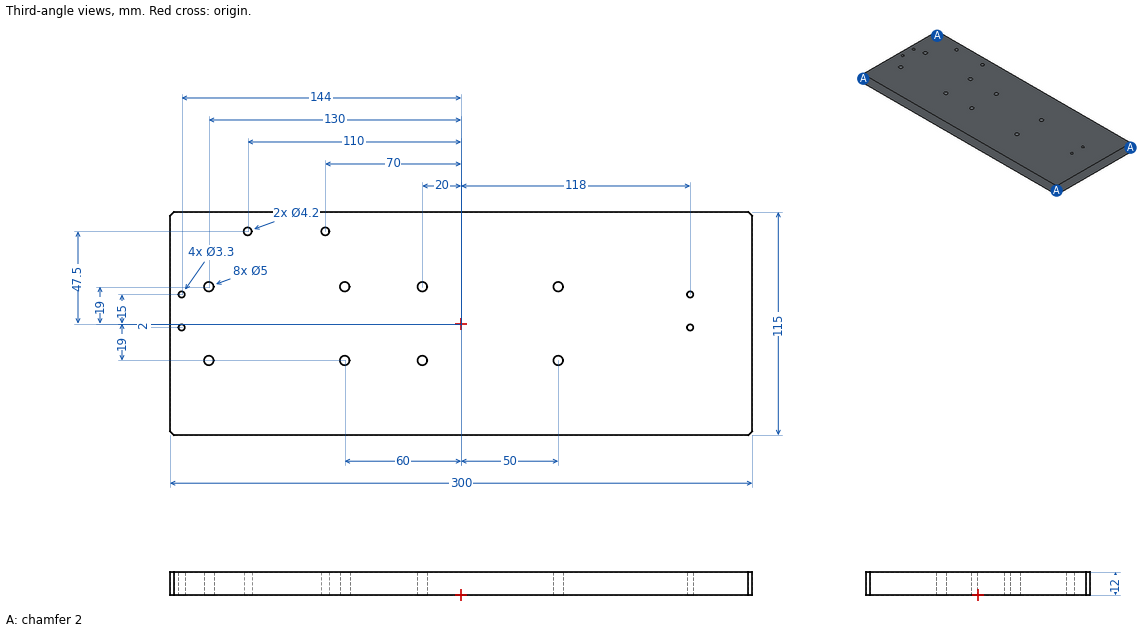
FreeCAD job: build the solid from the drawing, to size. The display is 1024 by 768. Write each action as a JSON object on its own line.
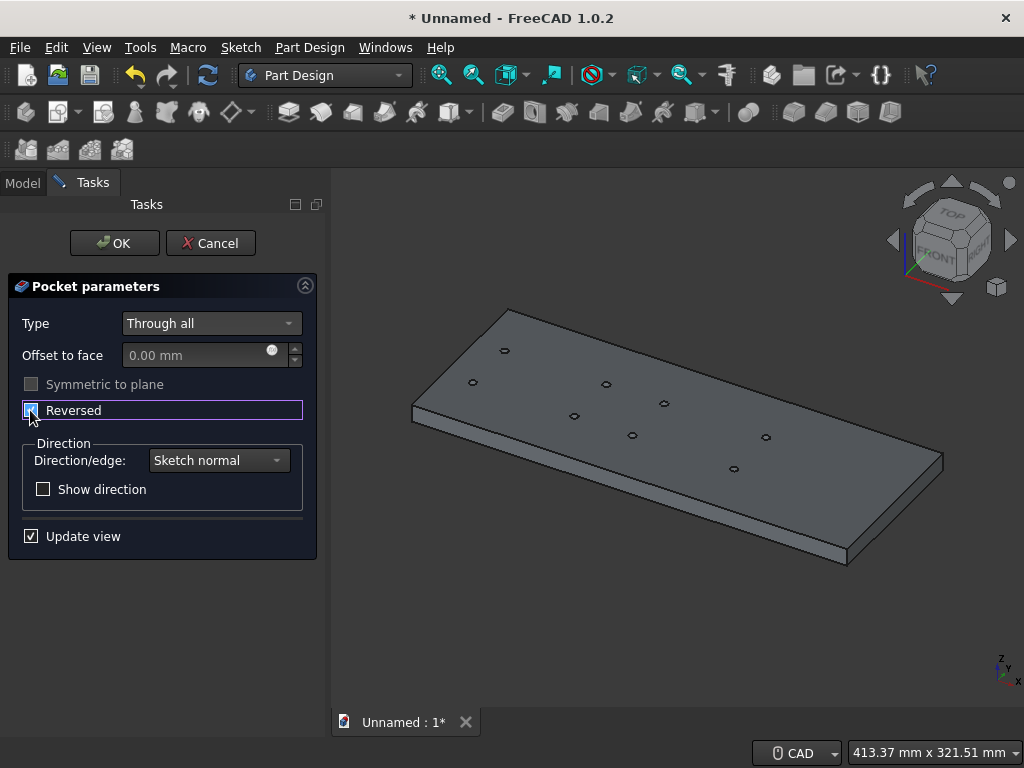
{"action": "left_click", "coordinate": [115, 243]}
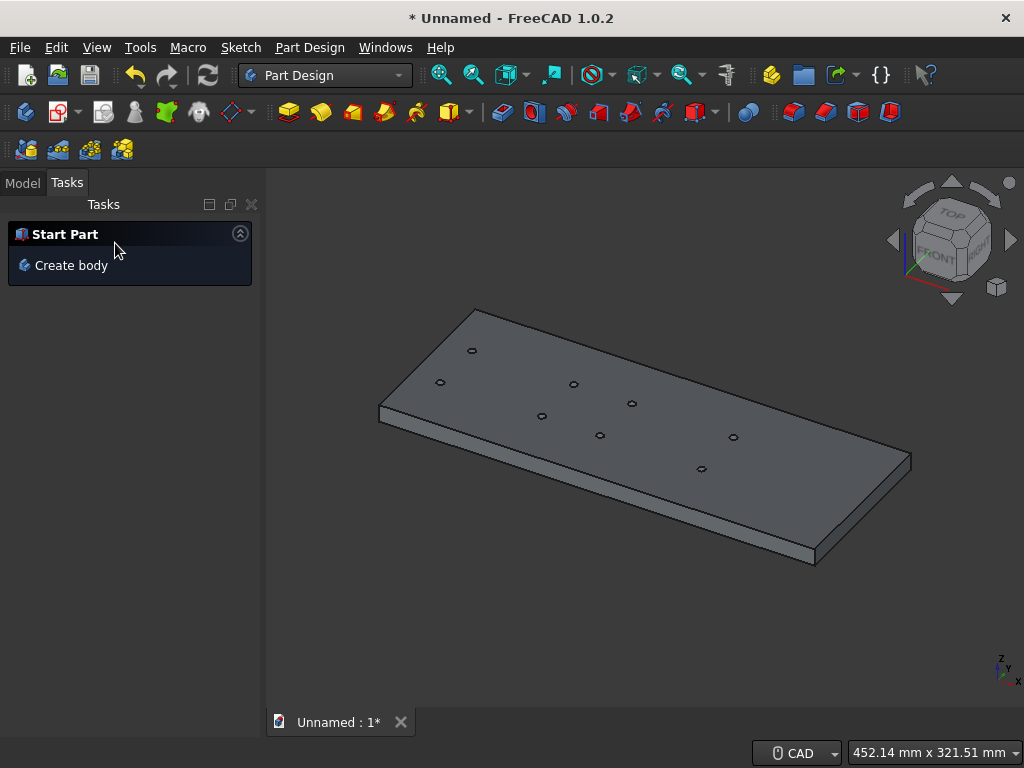
{"action": "left_click", "coordinate": [769, 469]}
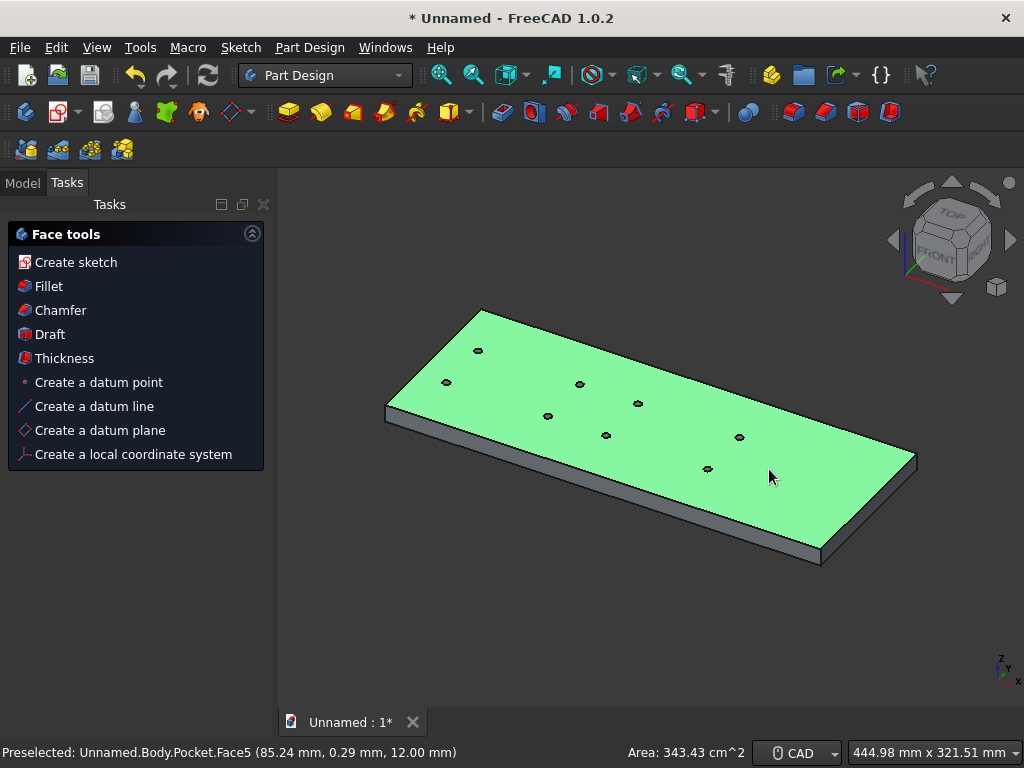
{"action": "left_click", "coordinate": [58, 112]}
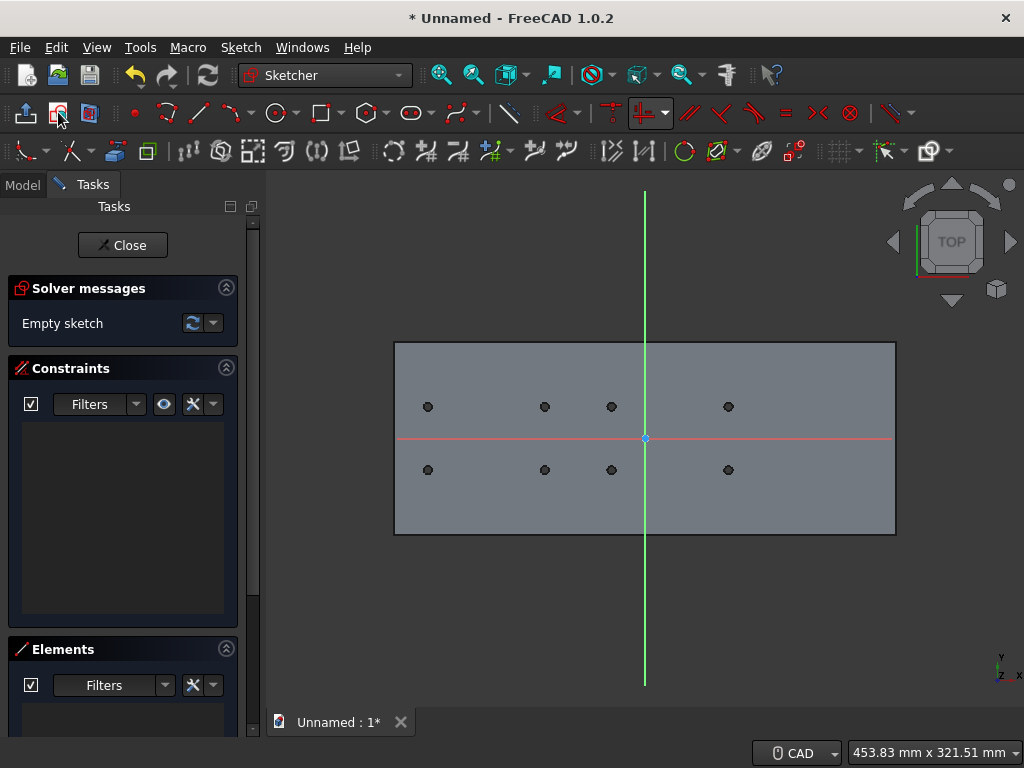
{"action": "scroll", "coordinate": [365, 488], "scroll_direction": "down", "scroll_amount": 1}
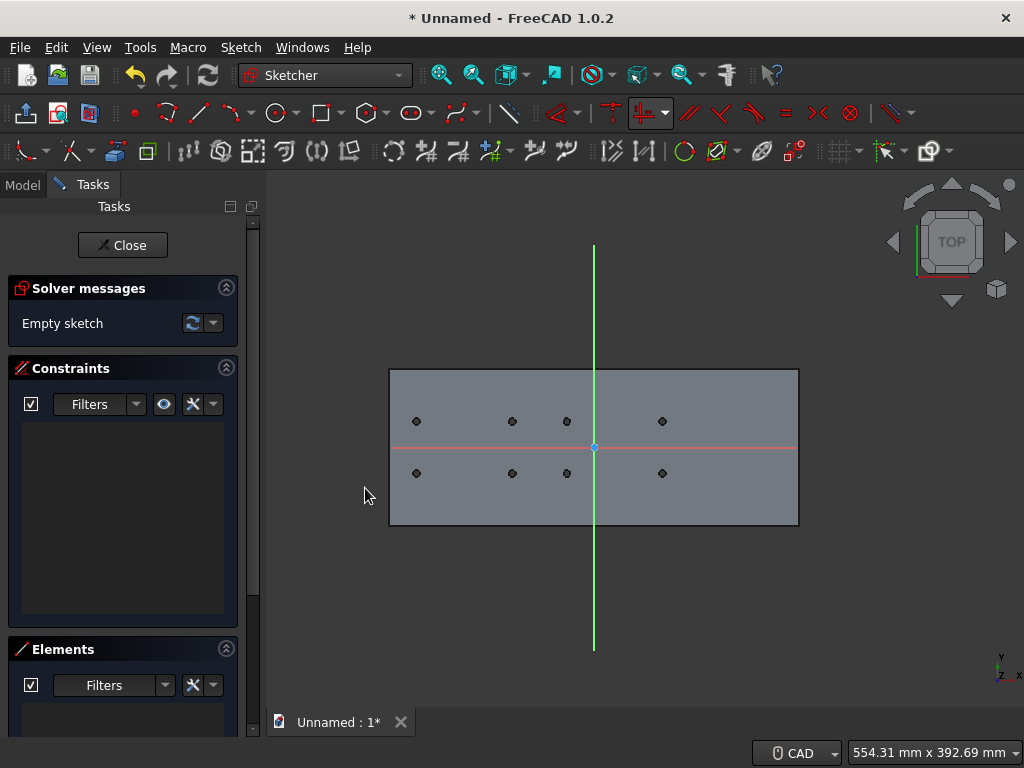
{"action": "key", "text": "g c"}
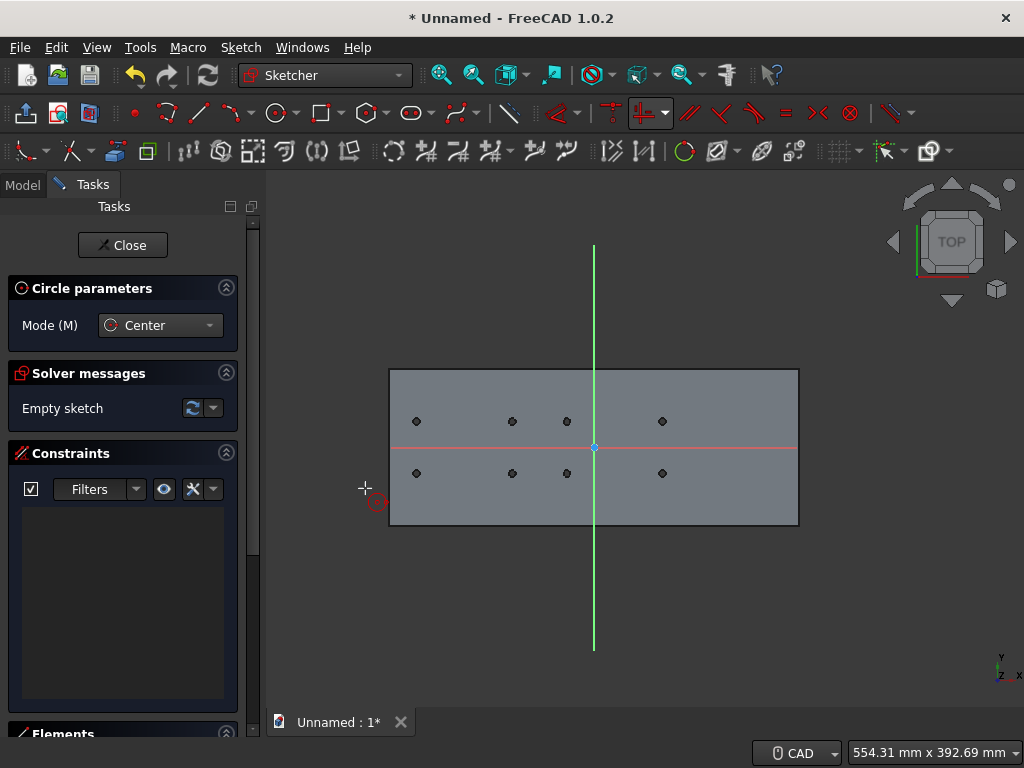
{"action": "scroll", "coordinate": [397, 427], "scroll_direction": "up", "scroll_amount": 12}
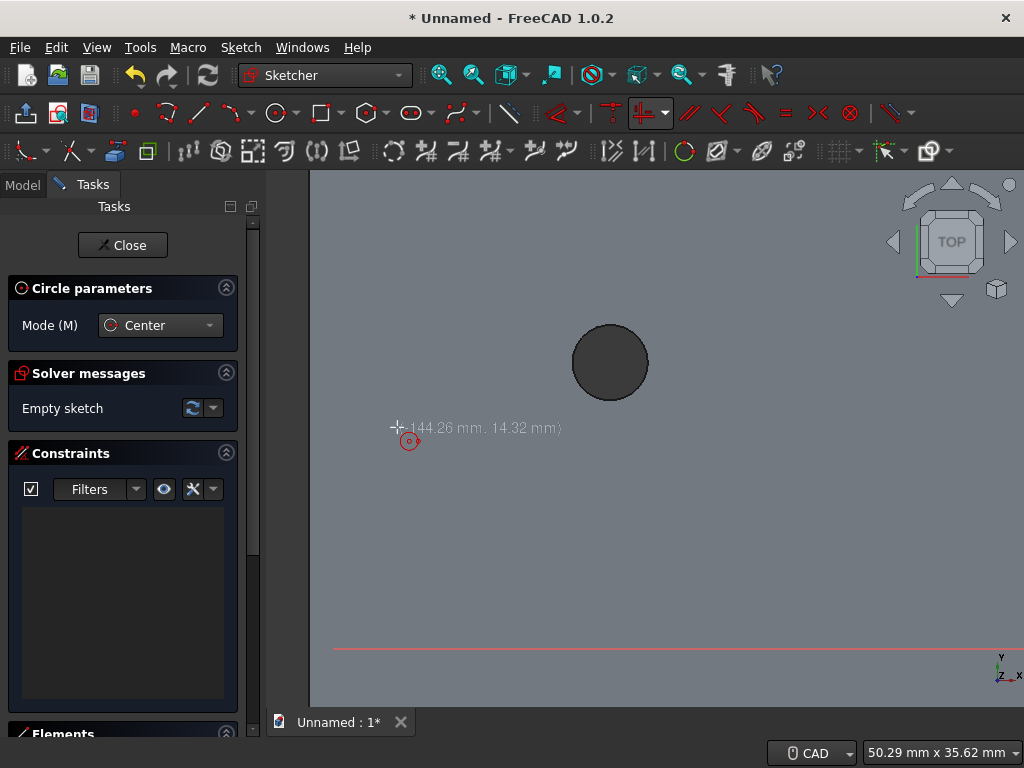
{"action": "scroll", "coordinate": [397, 427], "scroll_direction": "down", "scroll_amount": 12}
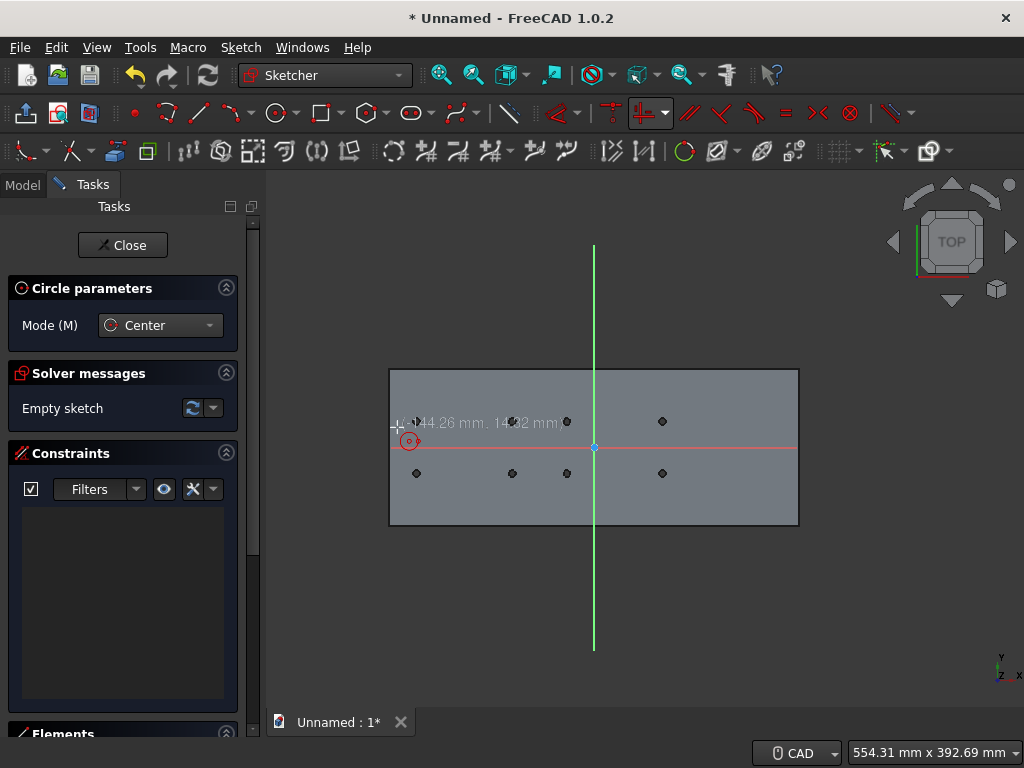
{"action": "left_click", "coordinate": [397, 427]}
{"action": "mouse_move", "coordinate": [399, 425]}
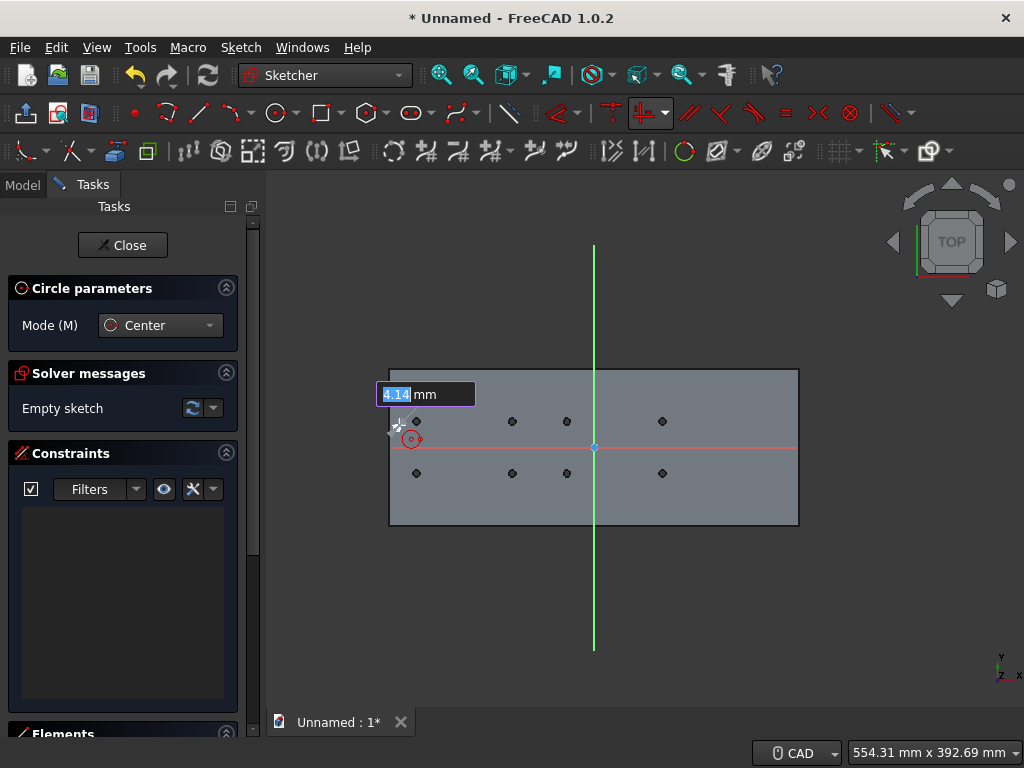
{"action": "type", "text": "3.3"}
{"action": "key", "text": "Return"}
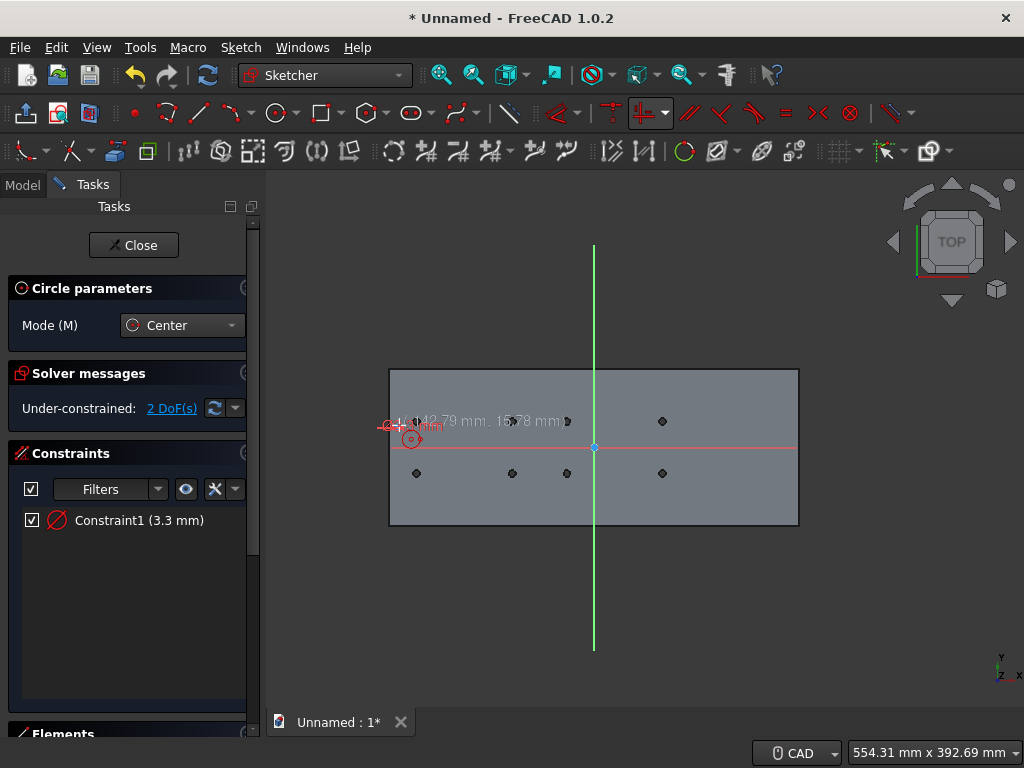
{"action": "scroll", "coordinate": [397, 450], "scroll_direction": "up", "scroll_amount": 12}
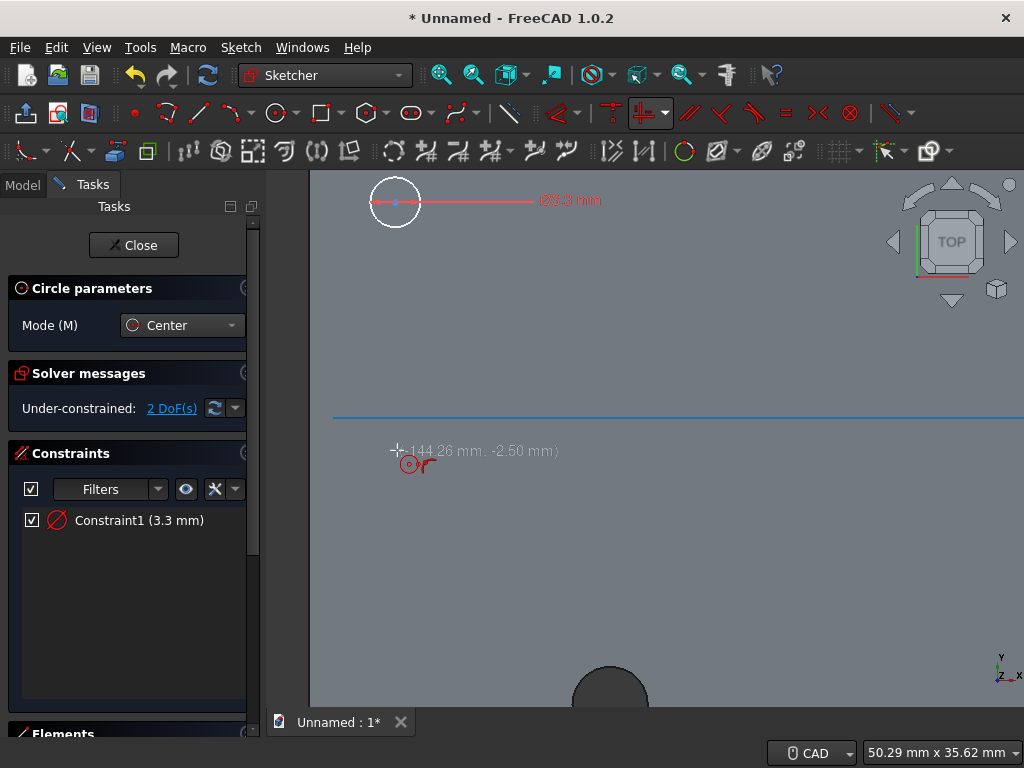
{"action": "left_click", "coordinate": [399, 448]}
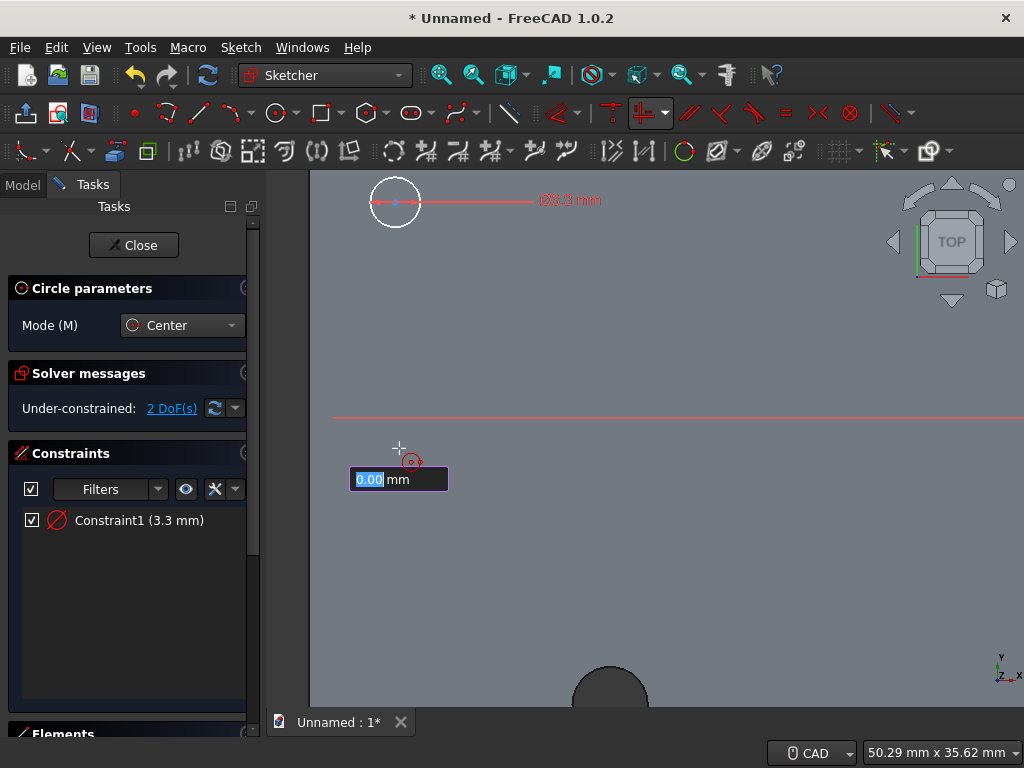
{"action": "scroll", "coordinate": [397, 450], "scroll_direction": "down", "scroll_amount": 12}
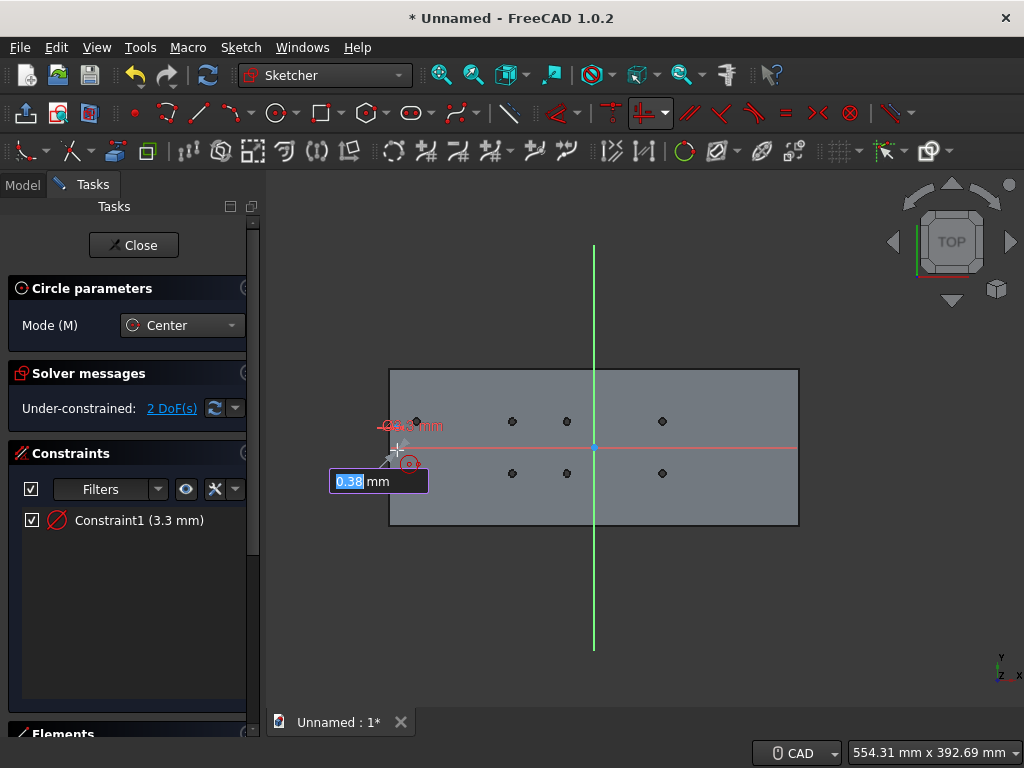
{"action": "scroll", "coordinate": [399, 452], "scroll_direction": "up", "scroll_amount": 7}
{"action": "mouse_move", "coordinate": [398, 450]}